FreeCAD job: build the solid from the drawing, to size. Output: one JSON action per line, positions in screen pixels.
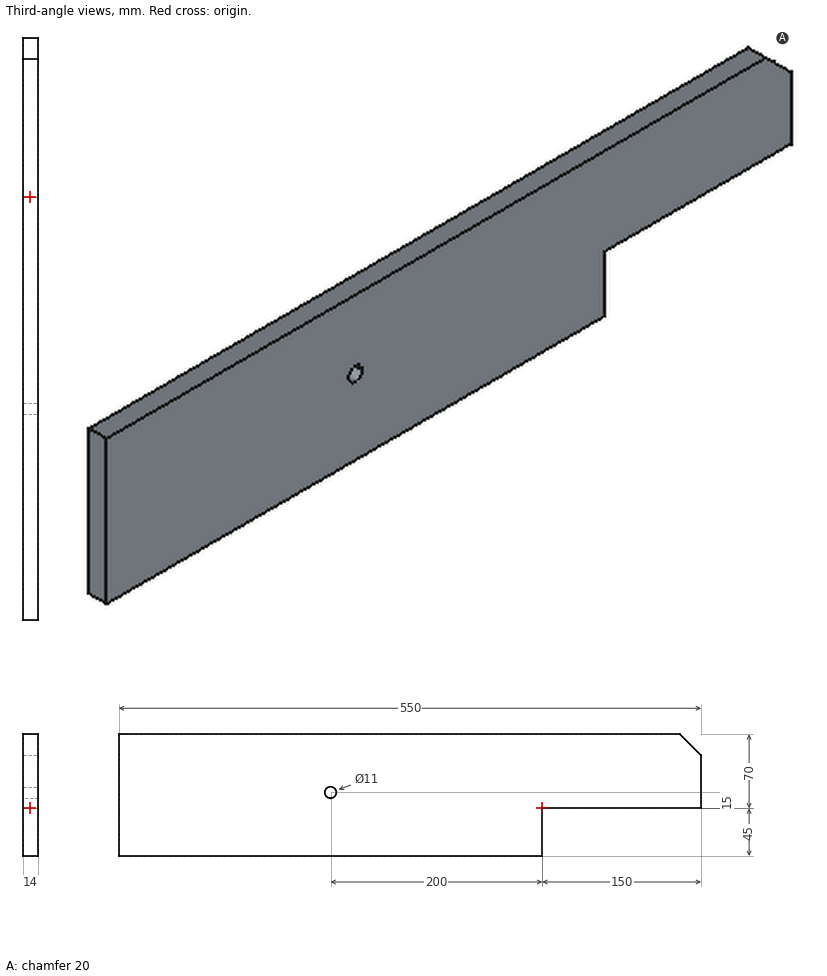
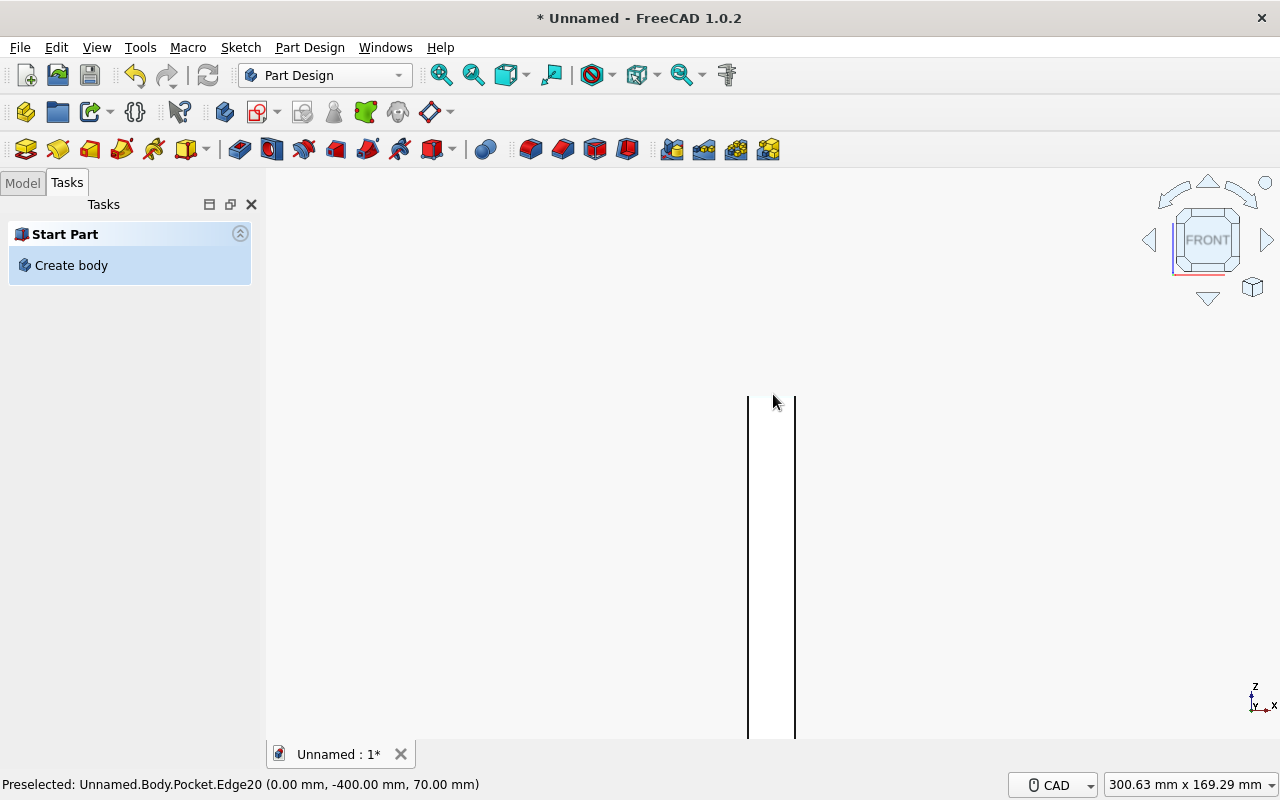
{"action": "left_click", "coordinate": [442, 76]}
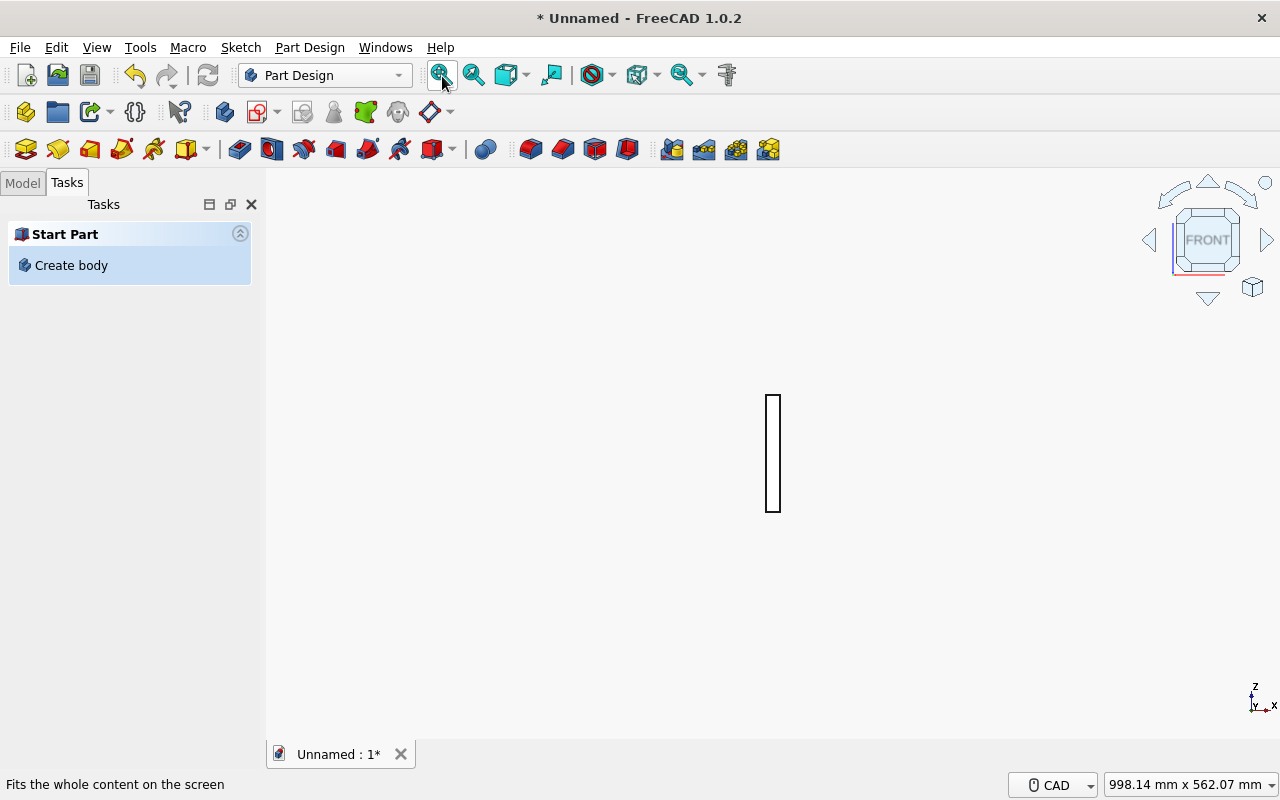
{"action": "key", "text": "3"}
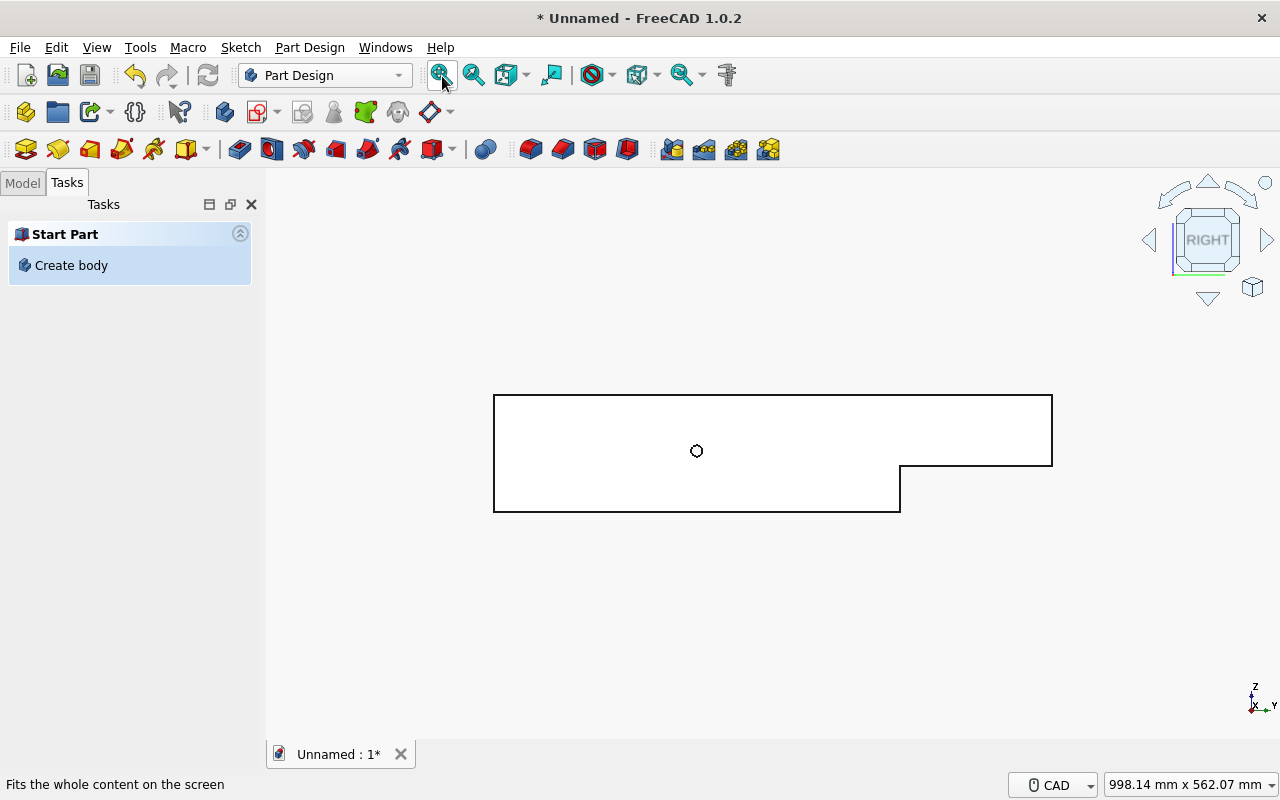
{"action": "scroll", "coordinate": [1052, 394], "scroll_direction": "up", "scroll_amount": 6}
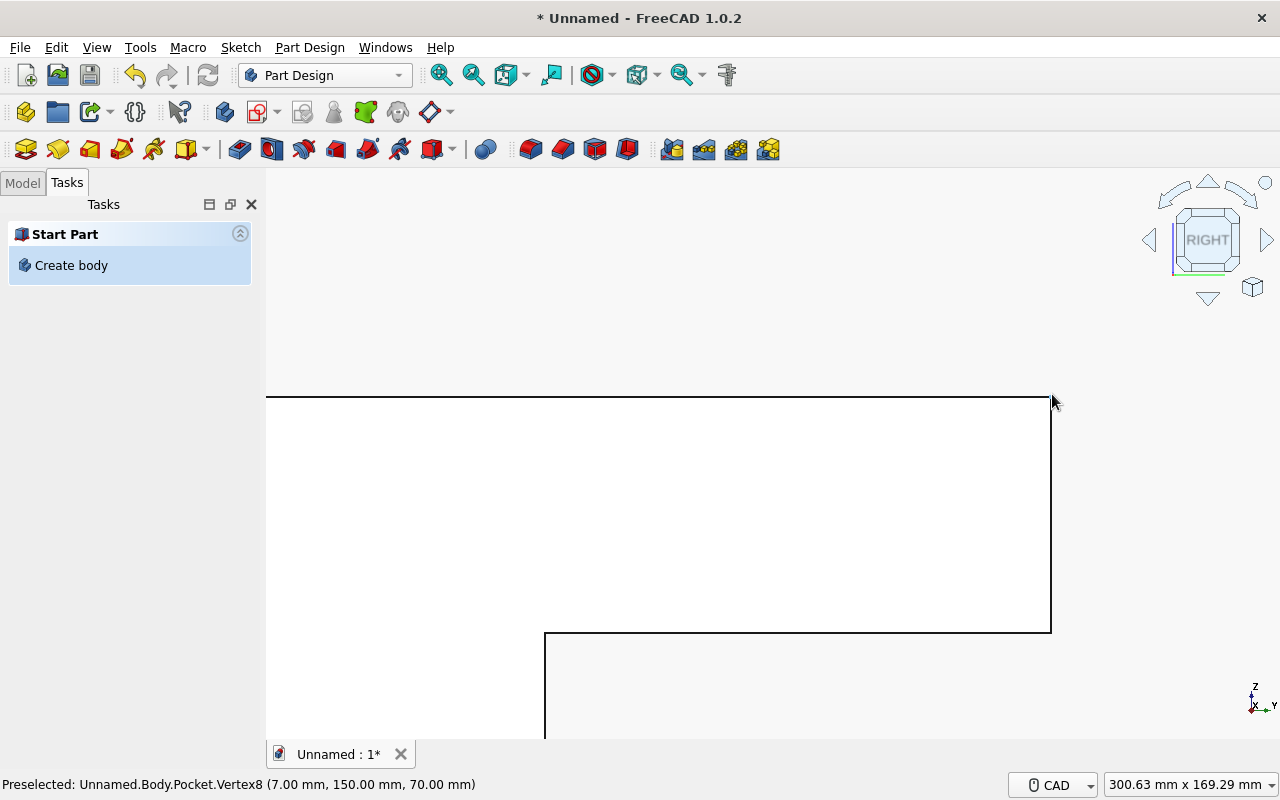
{"action": "left_click", "coordinate": [442, 76]}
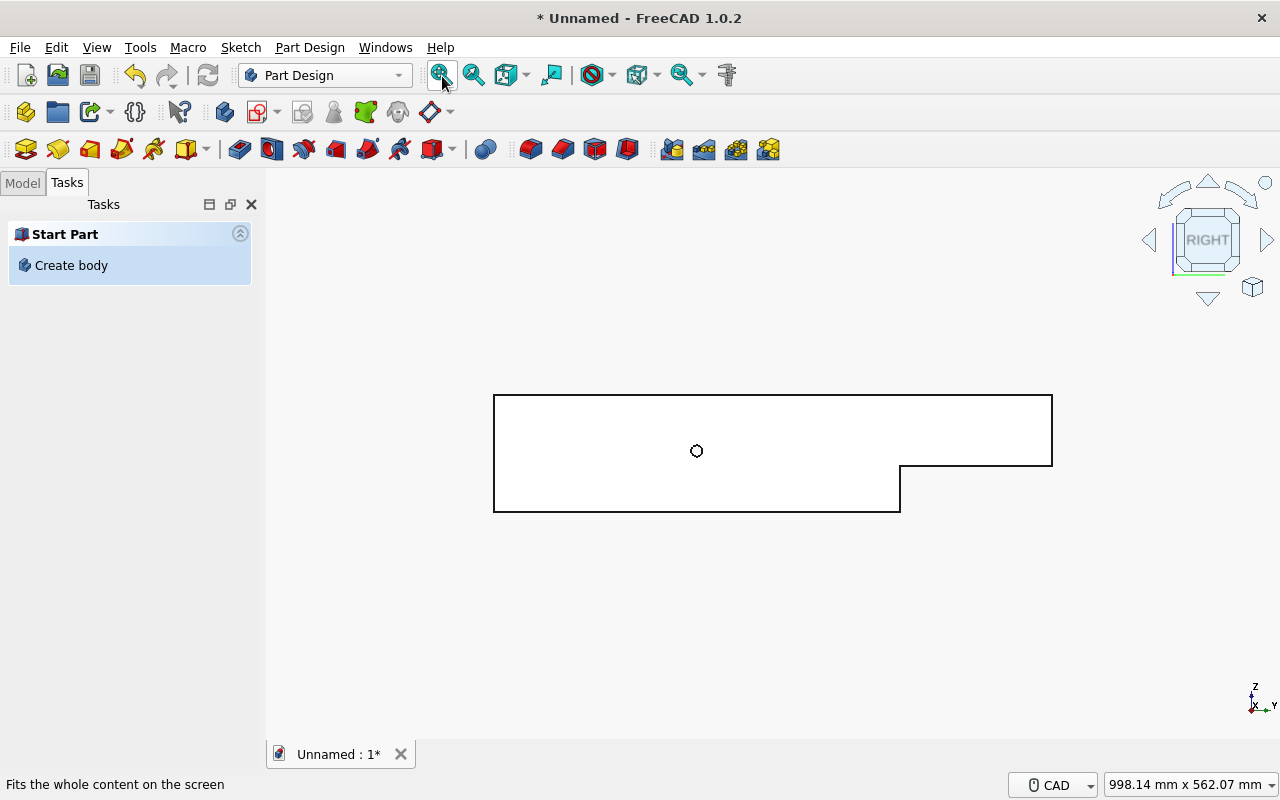
{"action": "key", "text": "5"}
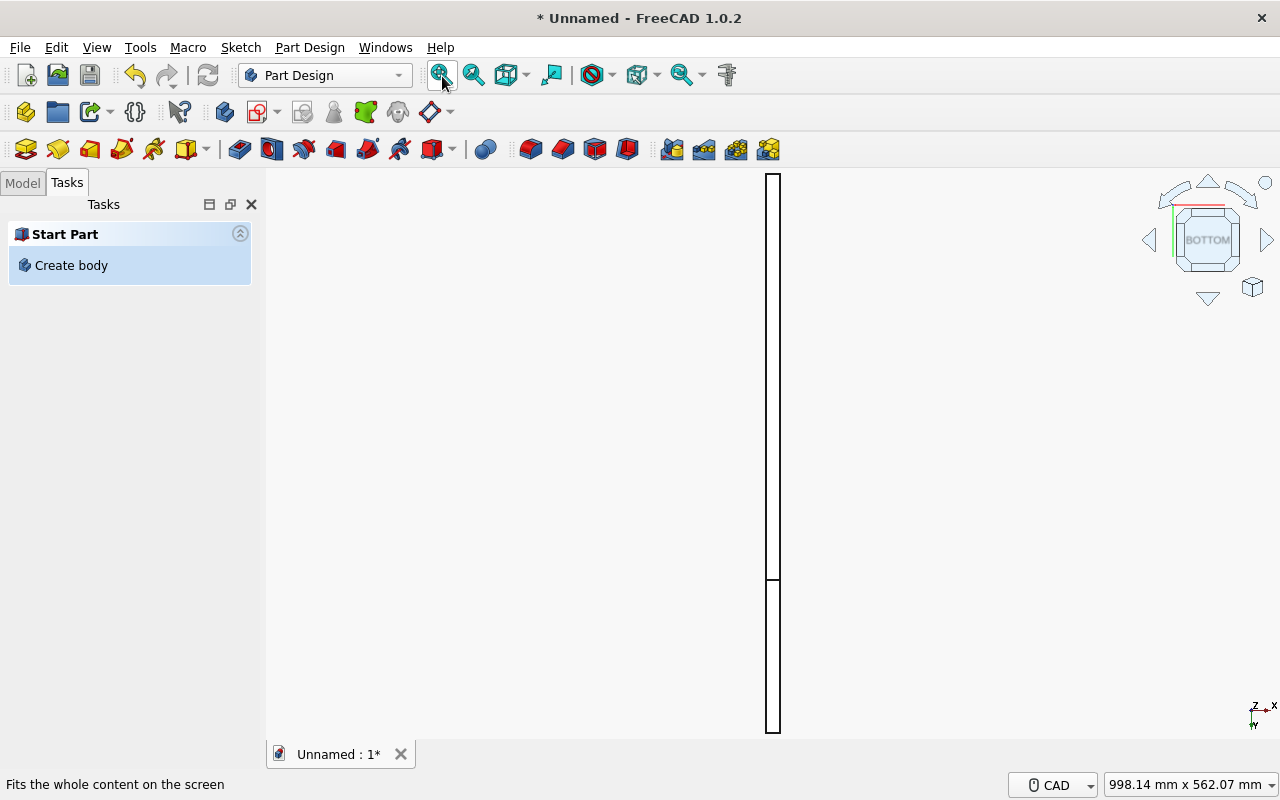
{"action": "key", "text": "4"}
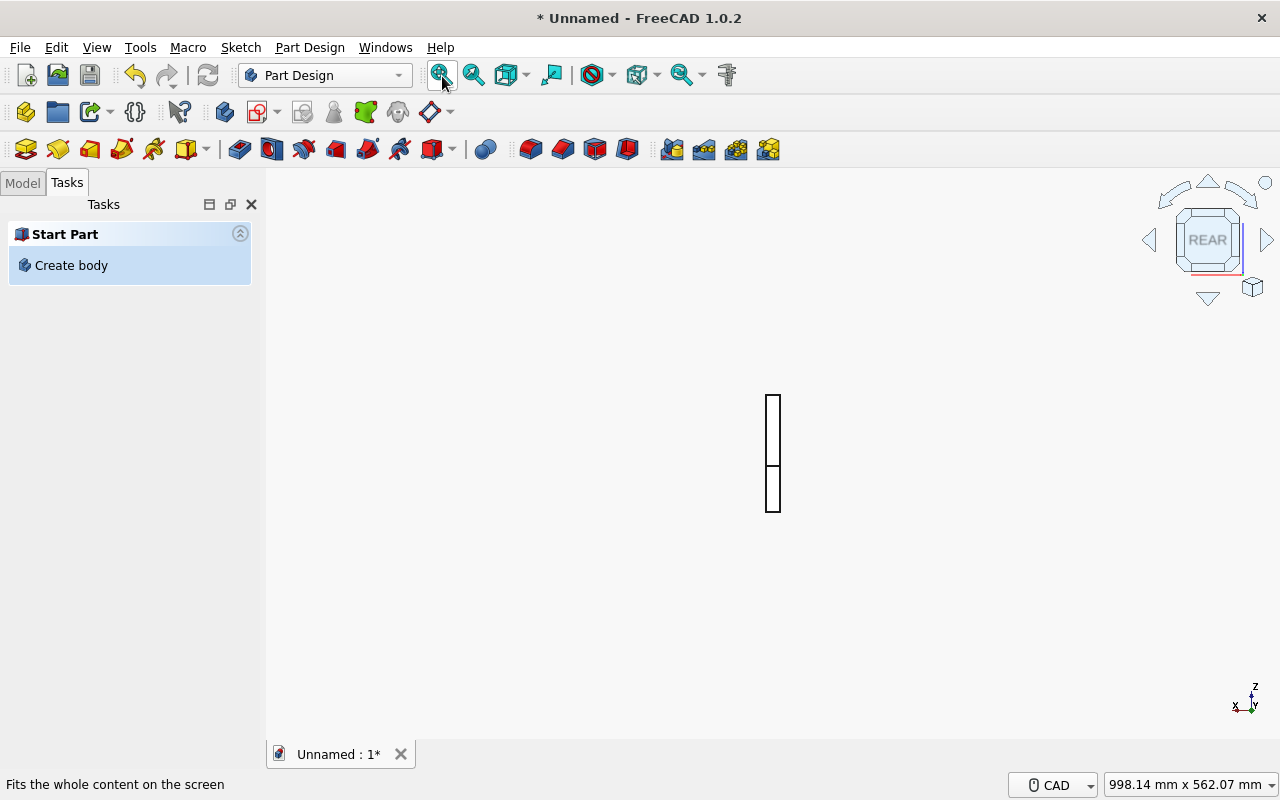
{"action": "left_click", "coordinate": [442, 76]}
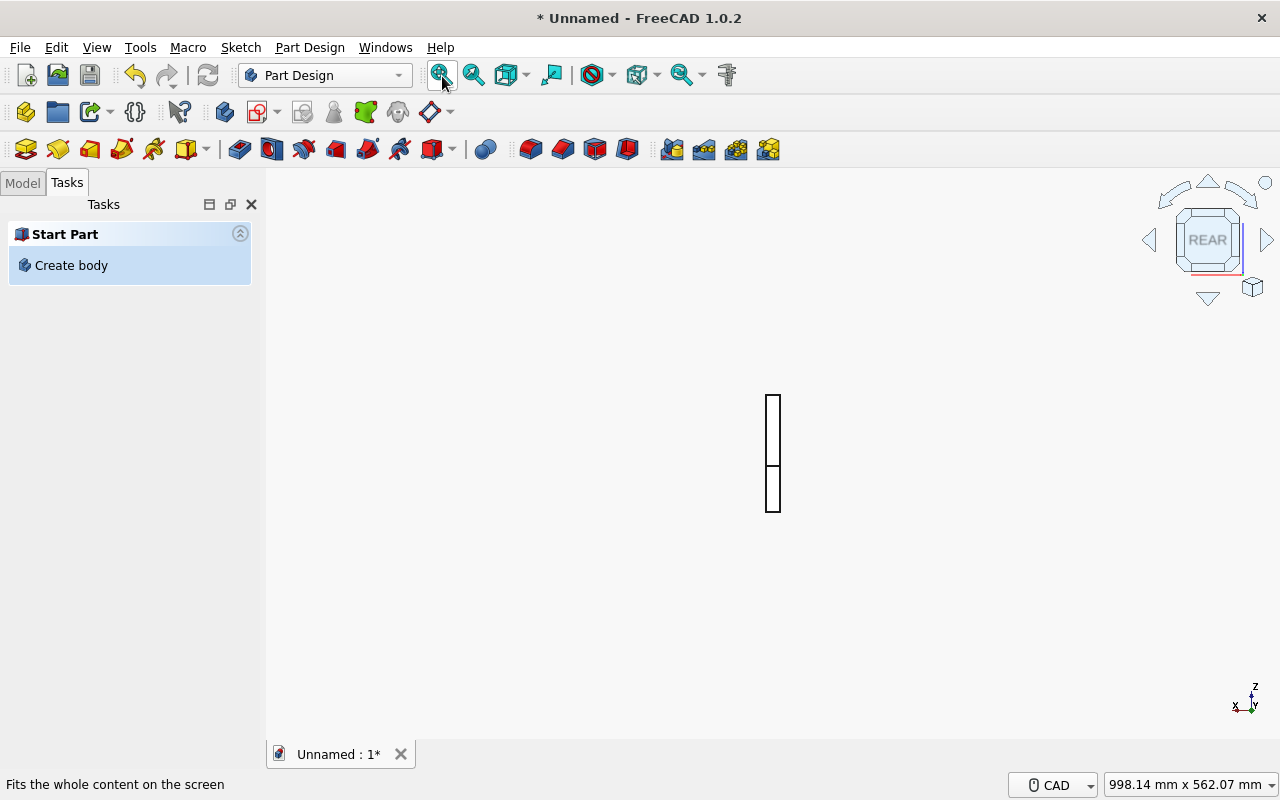
{"action": "left_click", "coordinate": [773, 394]}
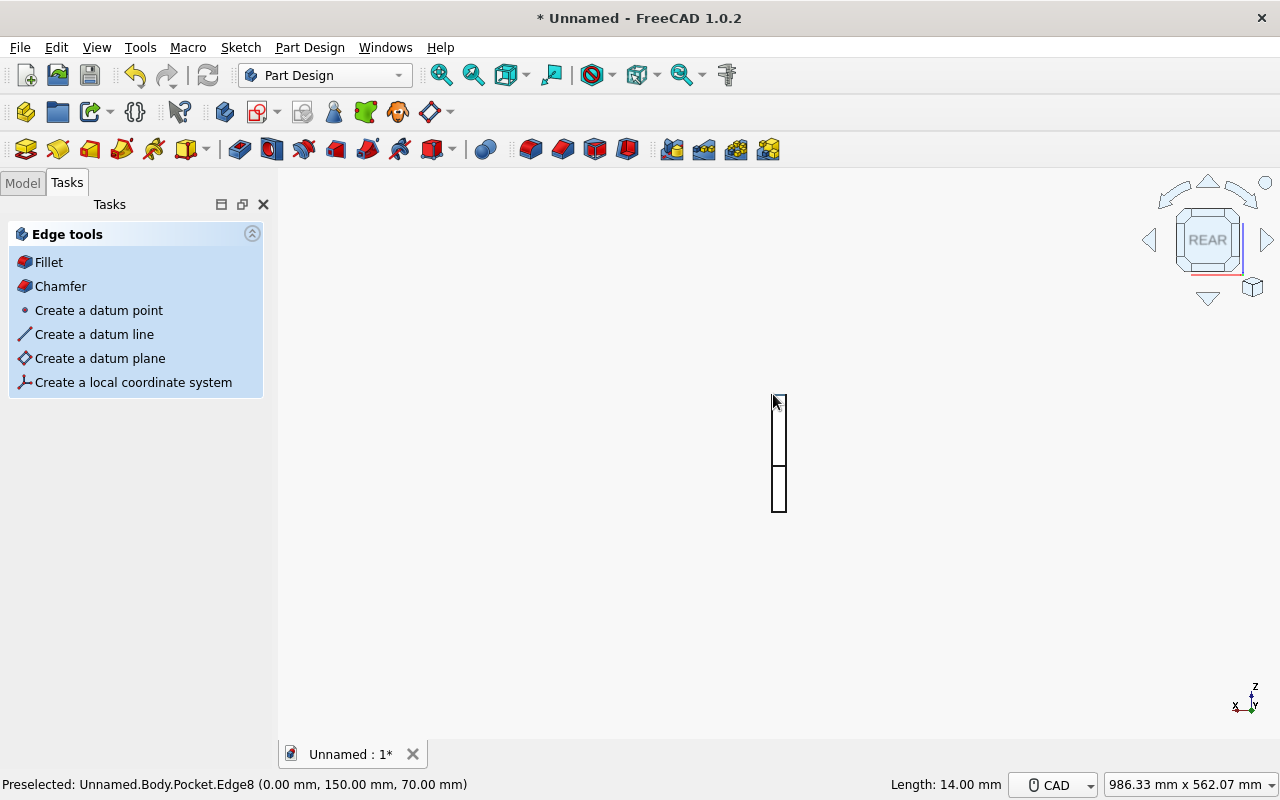
{"action": "left_click", "coordinate": [564, 150]}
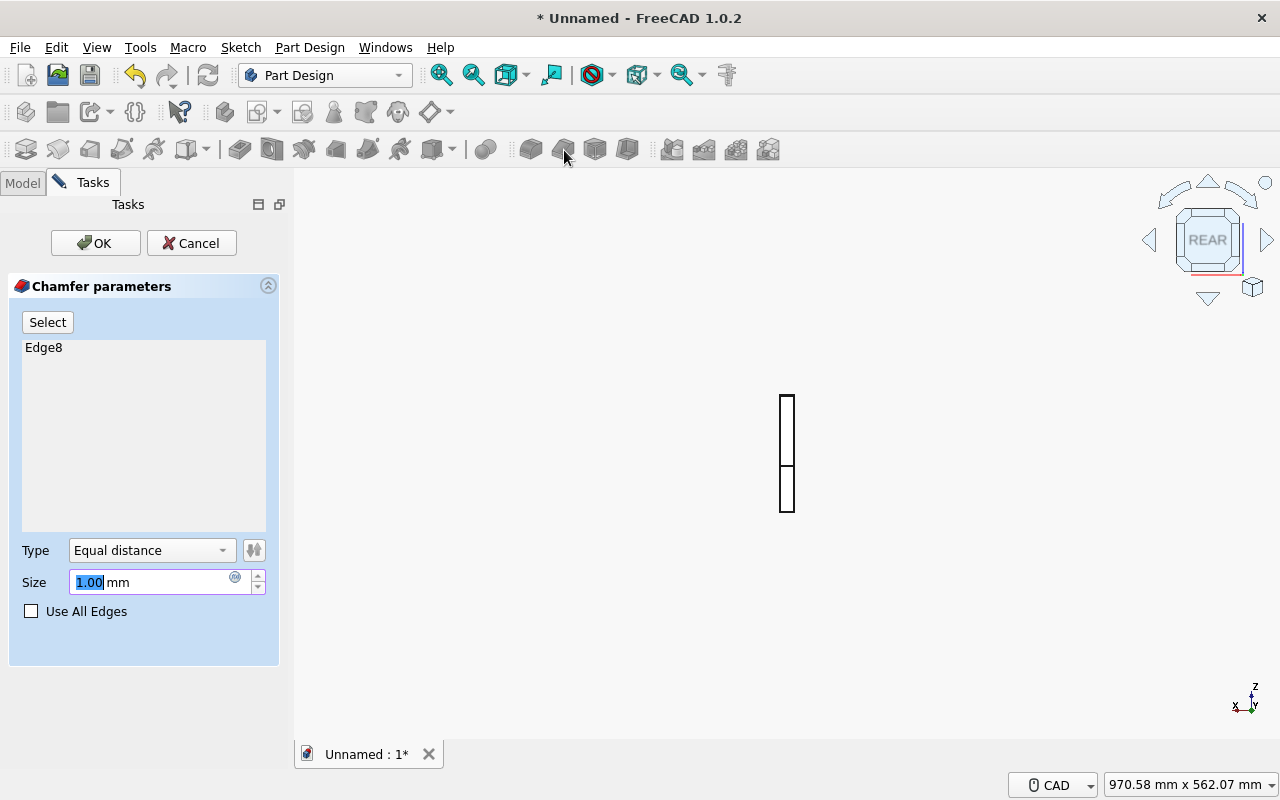
{"action": "type", "text": "20"}
{"action": "key", "text": "Tab"}